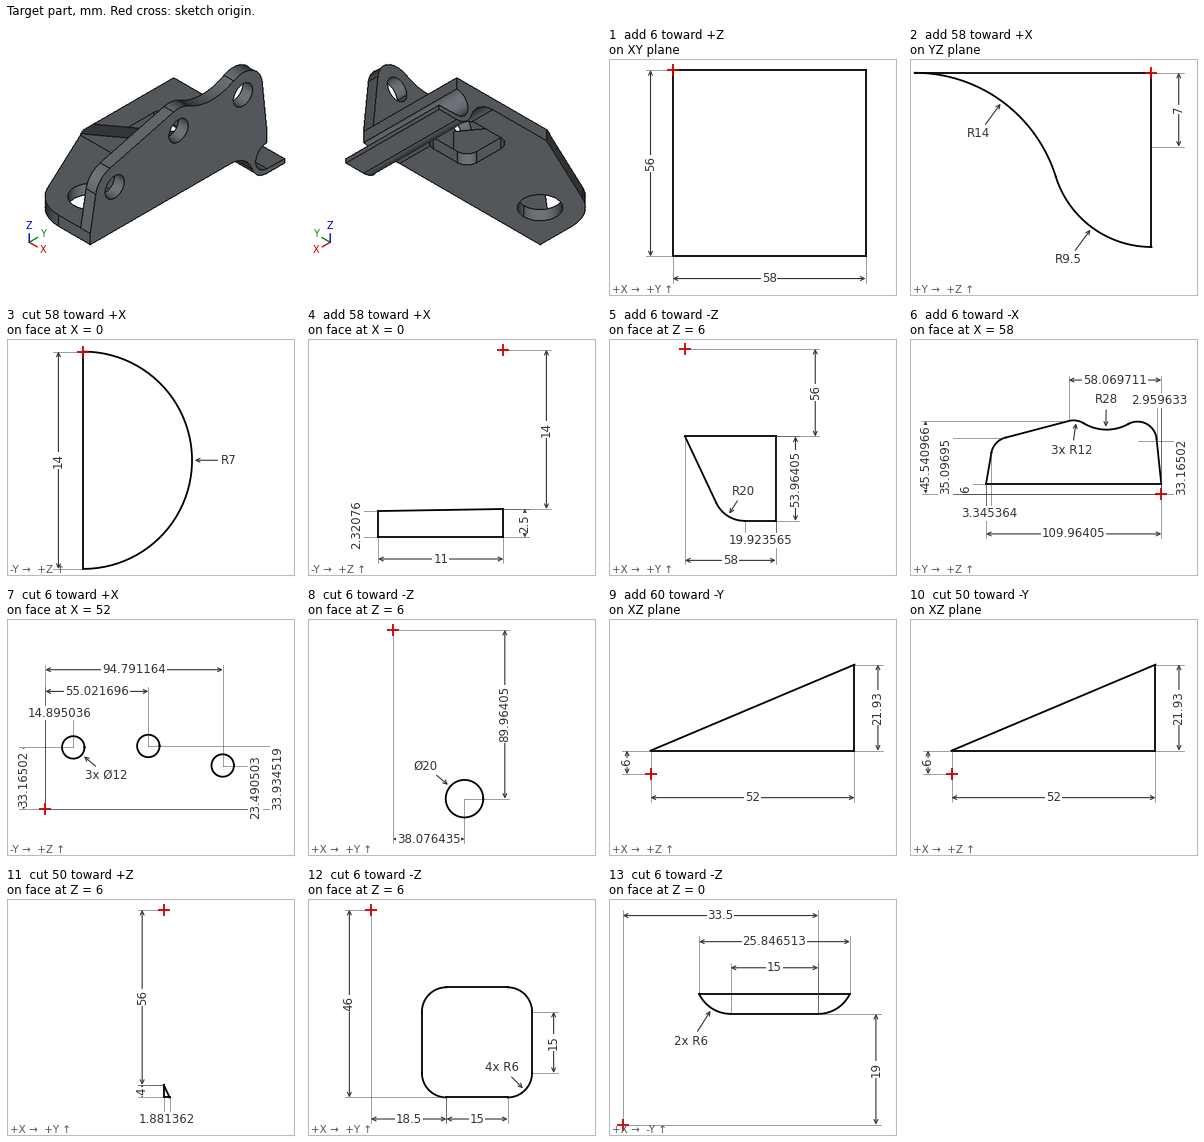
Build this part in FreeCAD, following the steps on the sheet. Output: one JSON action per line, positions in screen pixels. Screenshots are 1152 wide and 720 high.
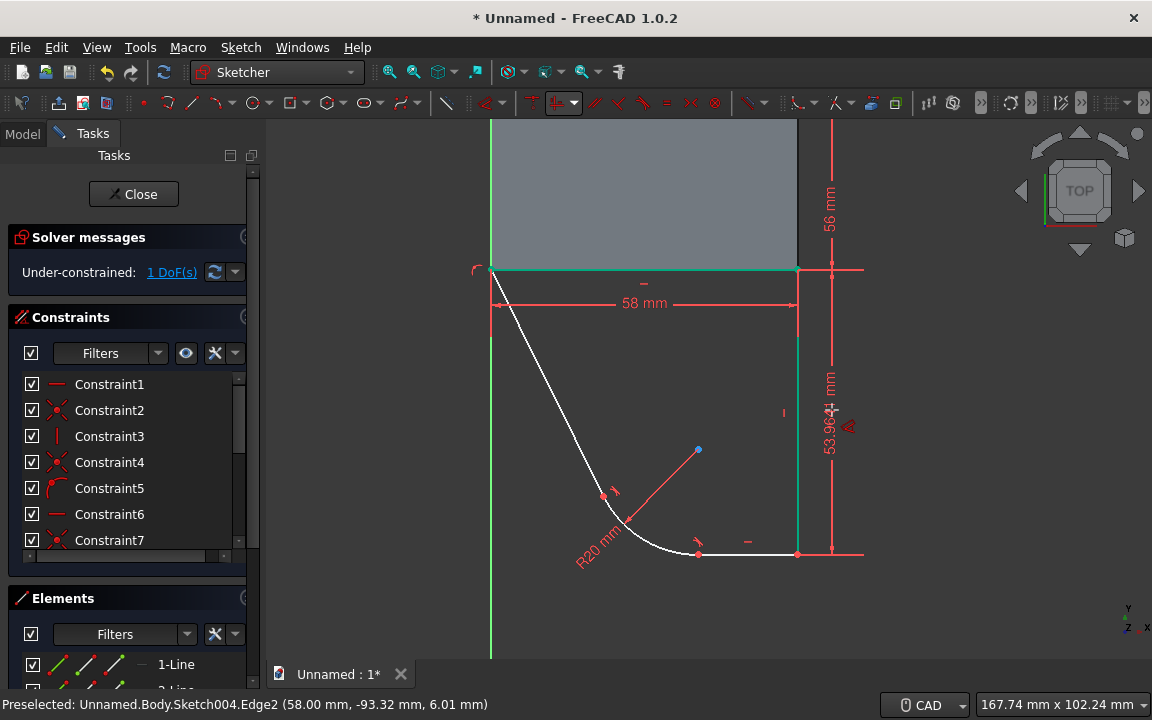
{"action": "left_click", "coordinate": [728, 555]}
{"action": "left_click", "coordinate": [748, 589]}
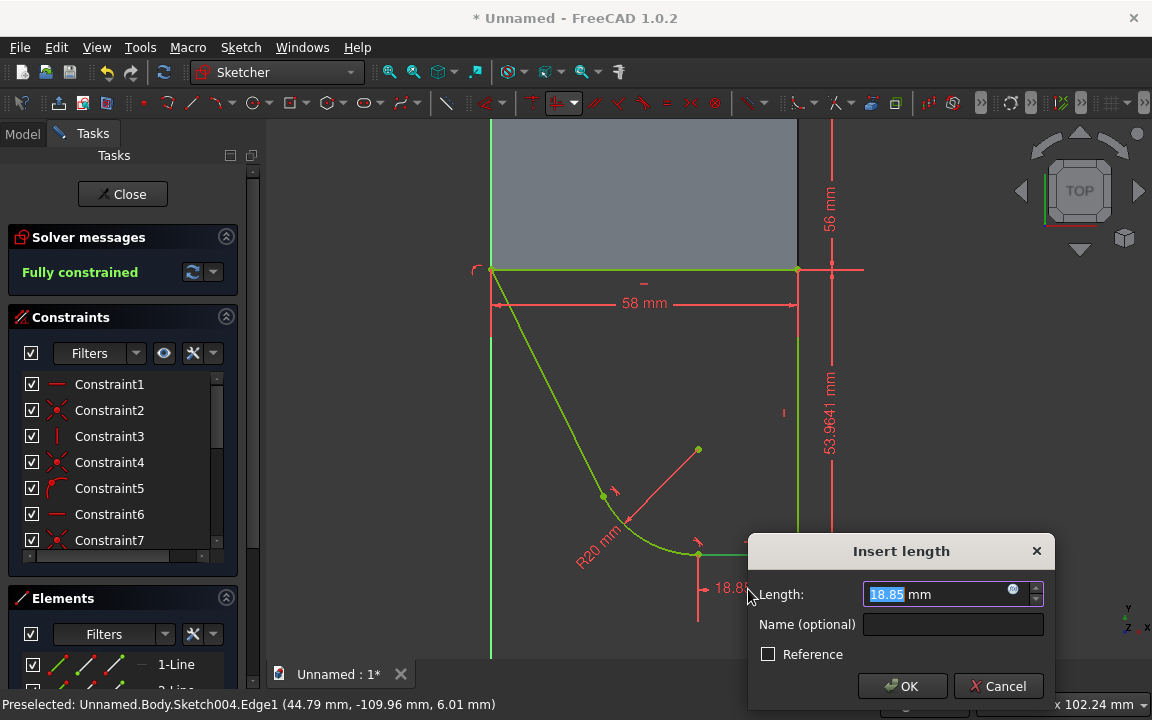
{"action": "type", "text": "19.923565"}
{"action": "key", "text": "Return"}
{"action": "key", "text": "Escape"}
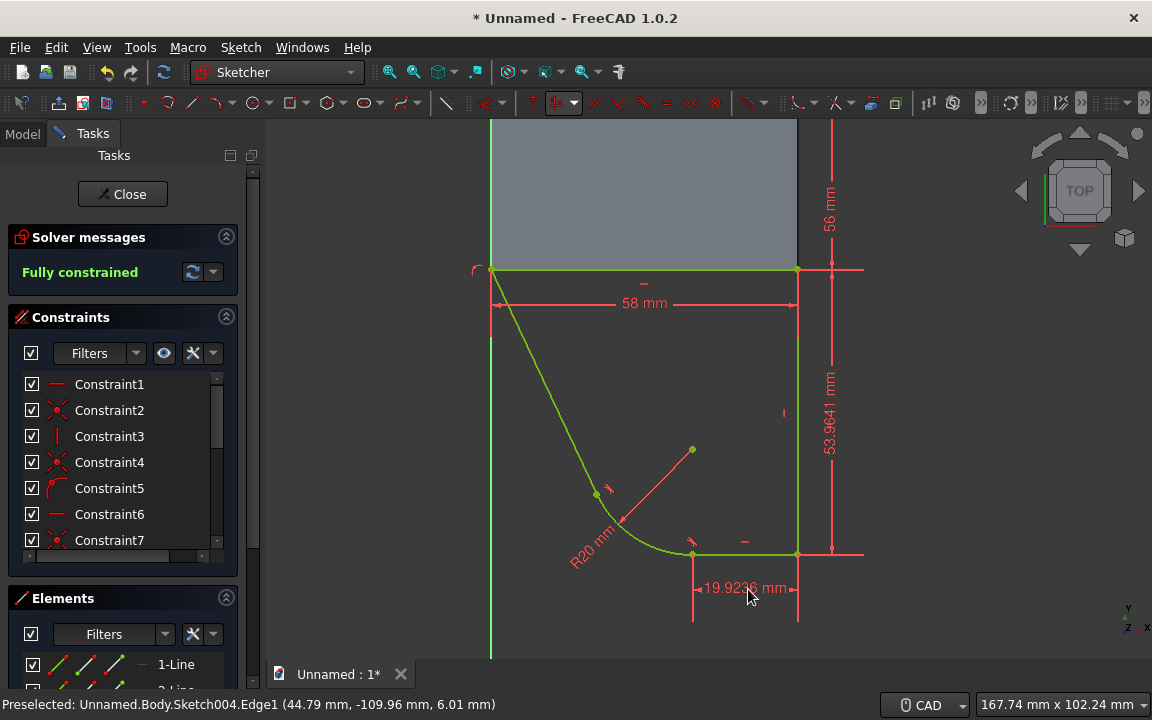
{"action": "left_click", "coordinate": [123, 194]}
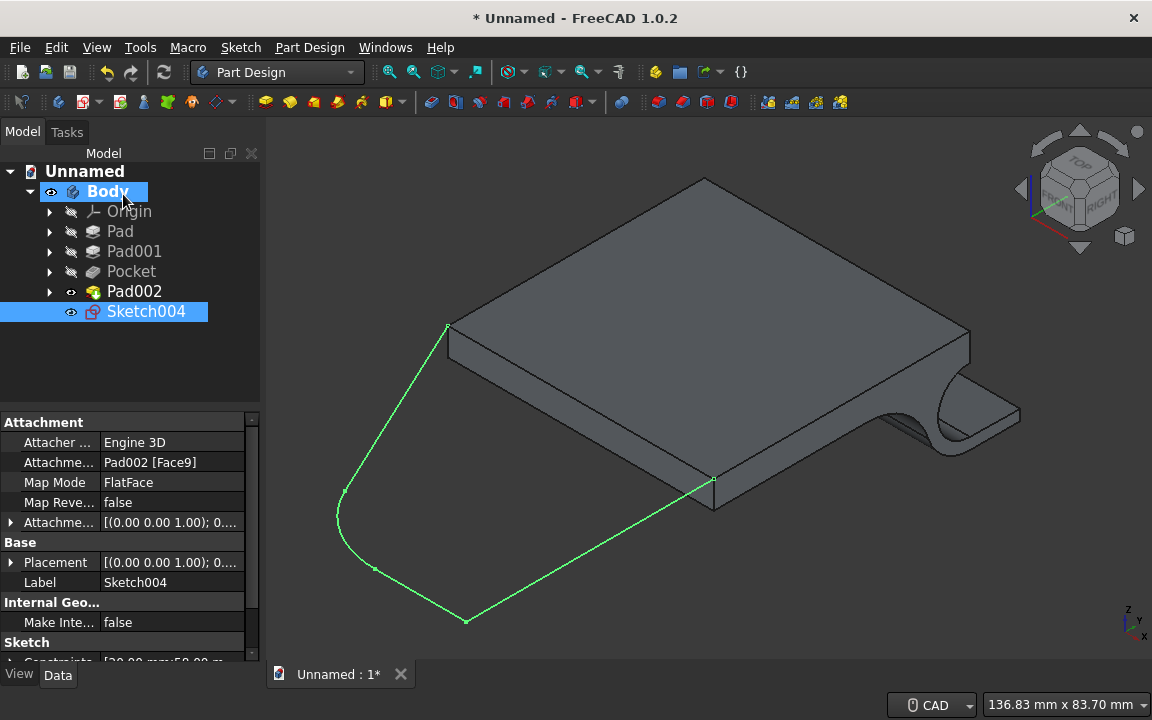
{"action": "left_click", "coordinate": [266, 102]}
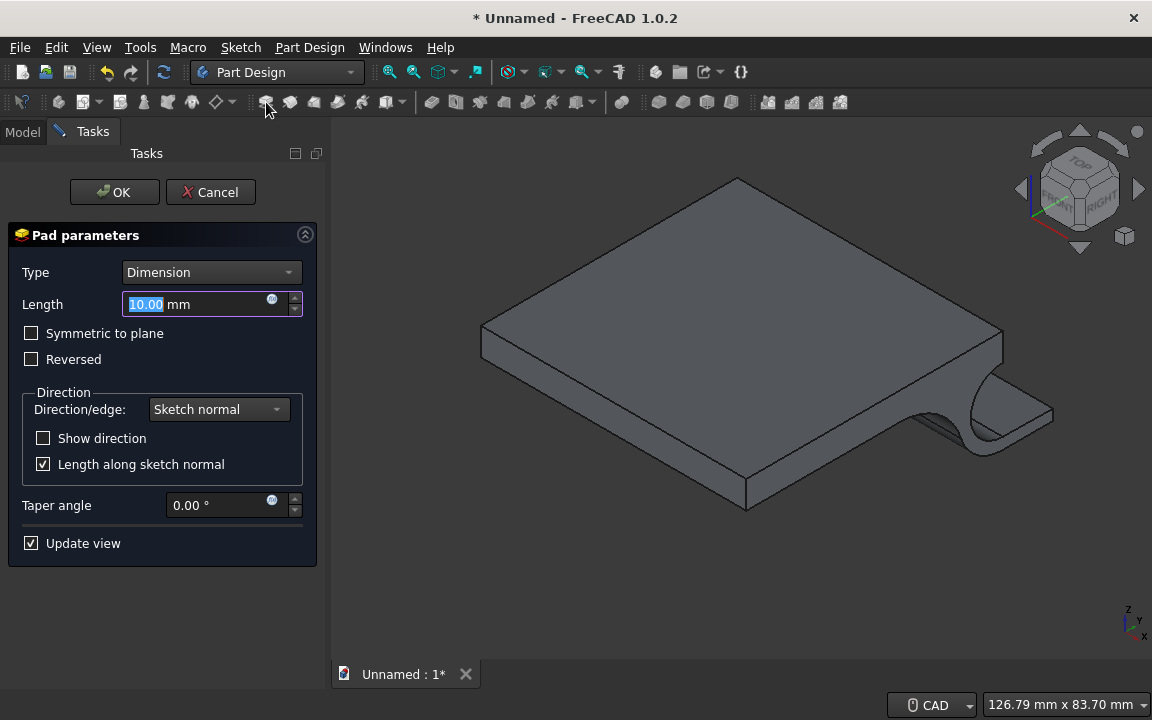
{"action": "type", "text": "6"}
{"action": "key", "text": "Tab"}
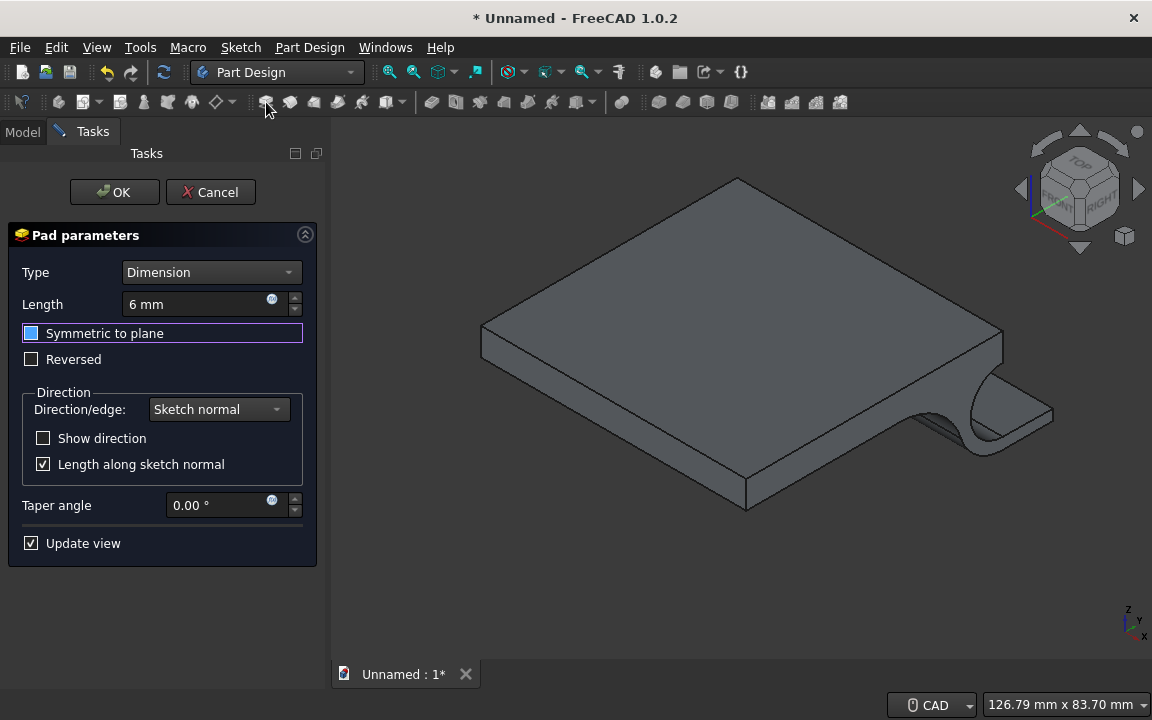
{"action": "left_click", "coordinate": [30, 359]}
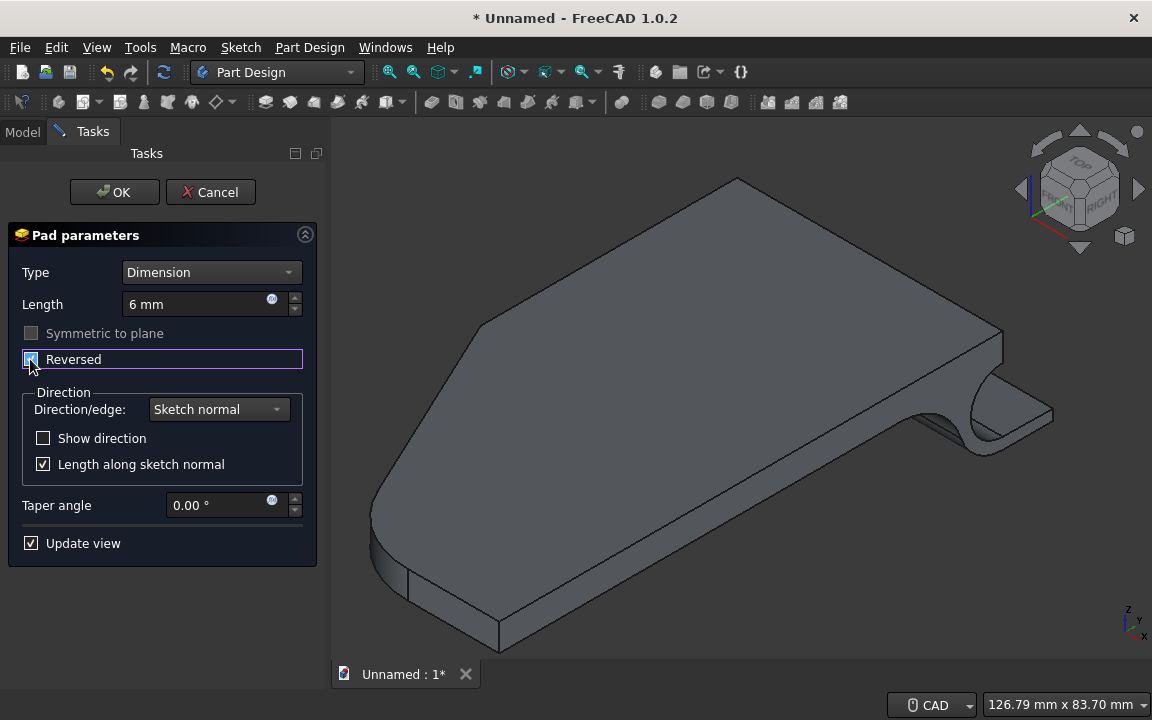
{"action": "left_click", "coordinate": [115, 192]}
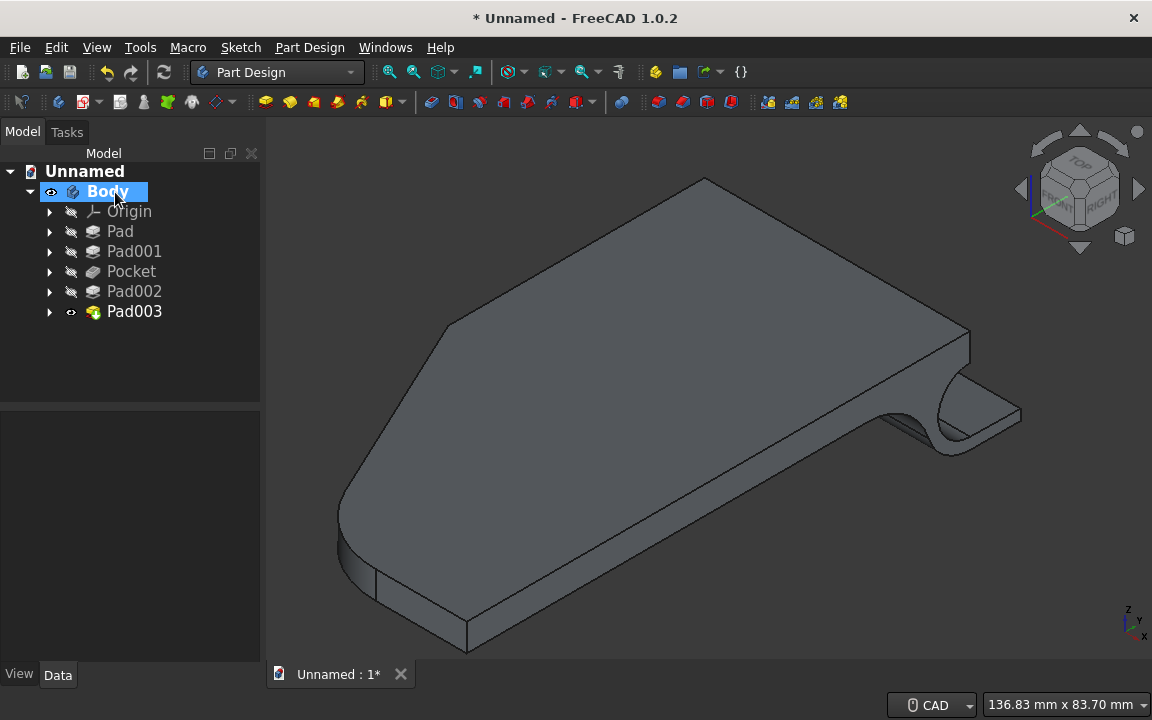
{"action": "left_click", "coordinate": [390, 72]}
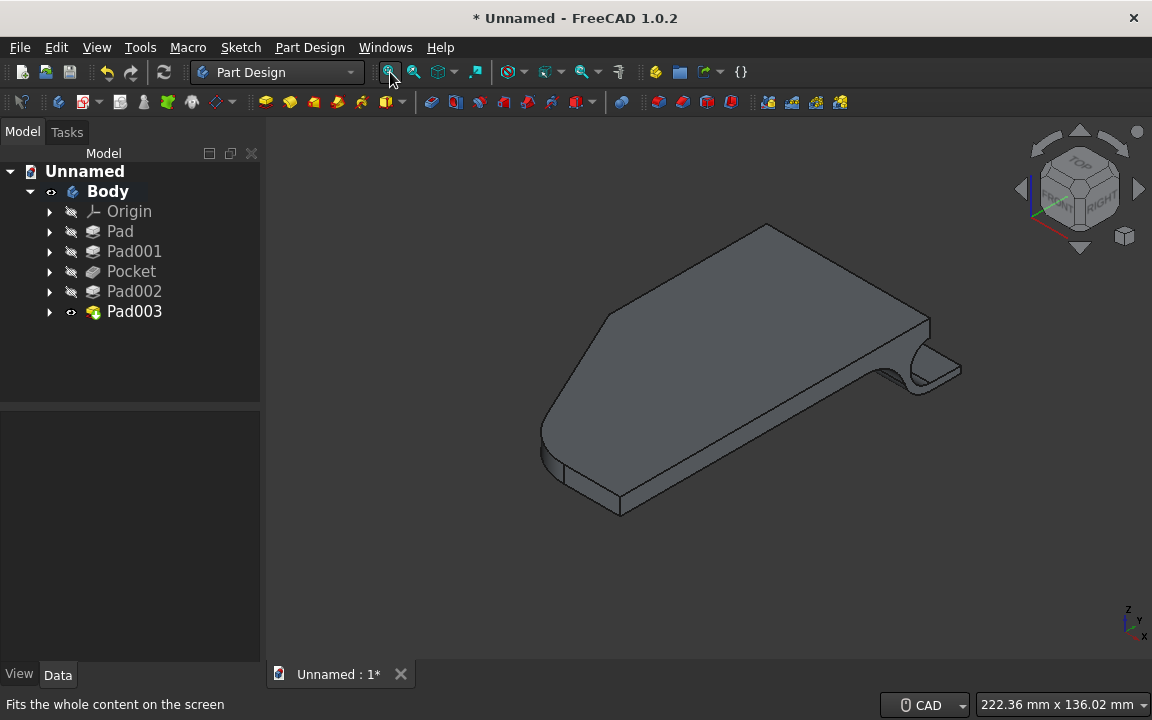
{"action": "left_click", "coordinate": [888, 357]}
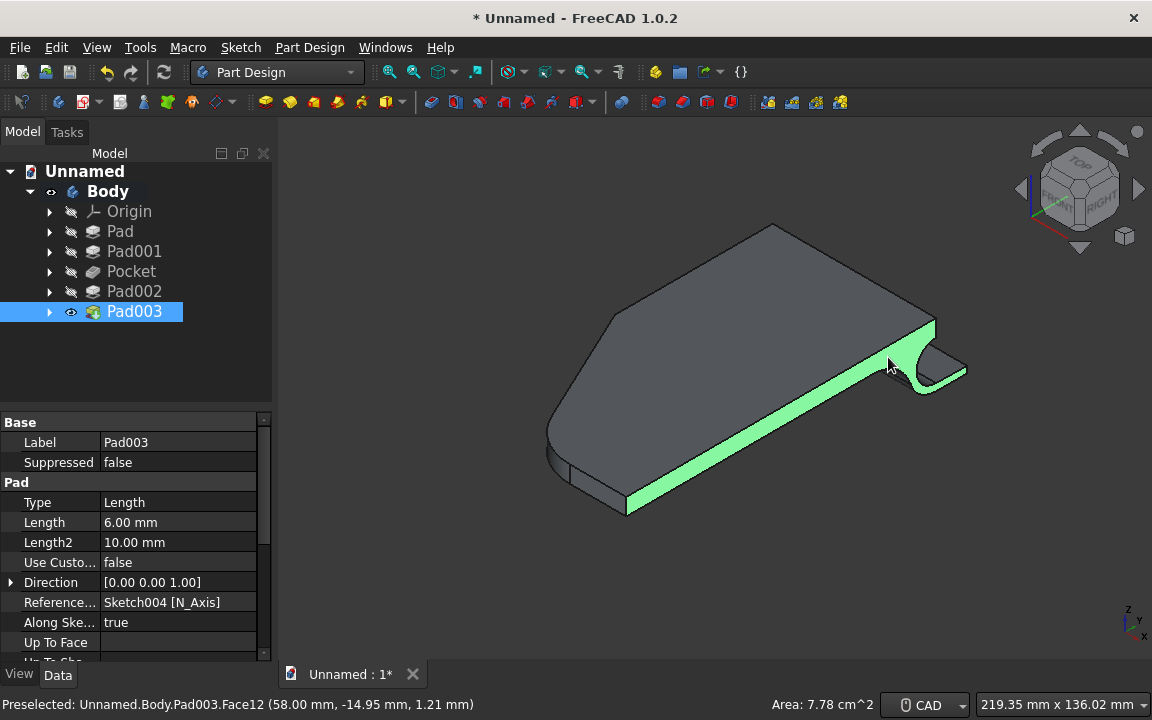
{"action": "left_click", "coordinate": [84, 102]}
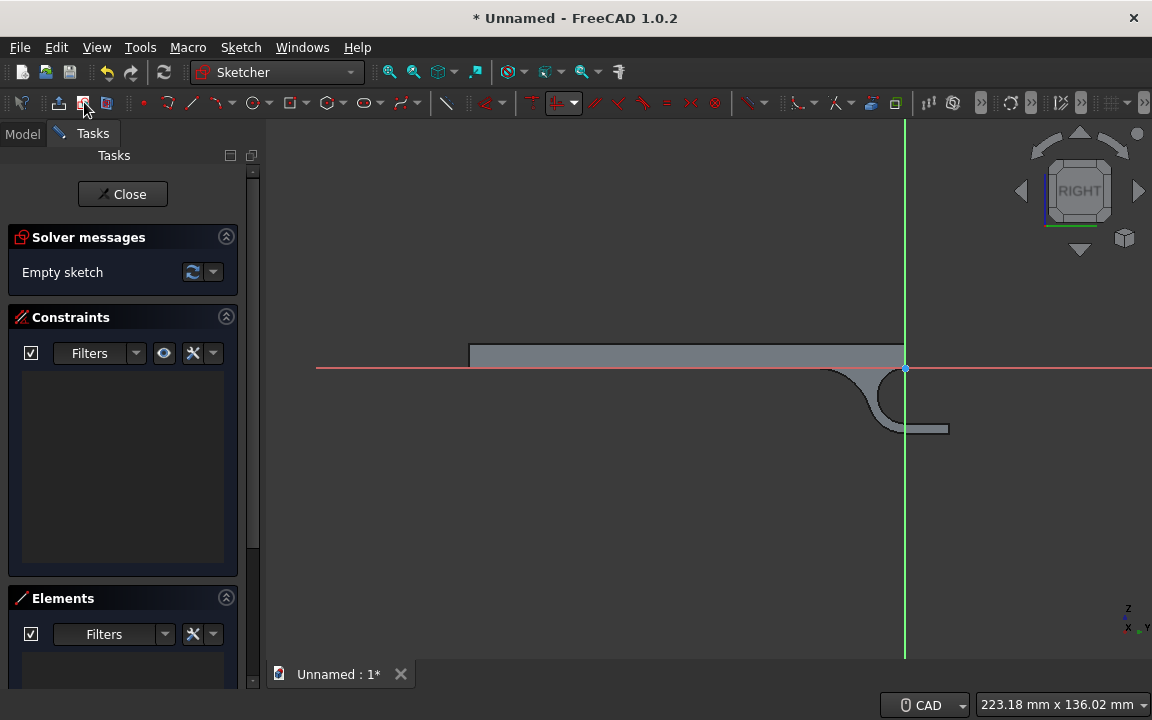
{"action": "left_click", "coordinate": [168, 104]}